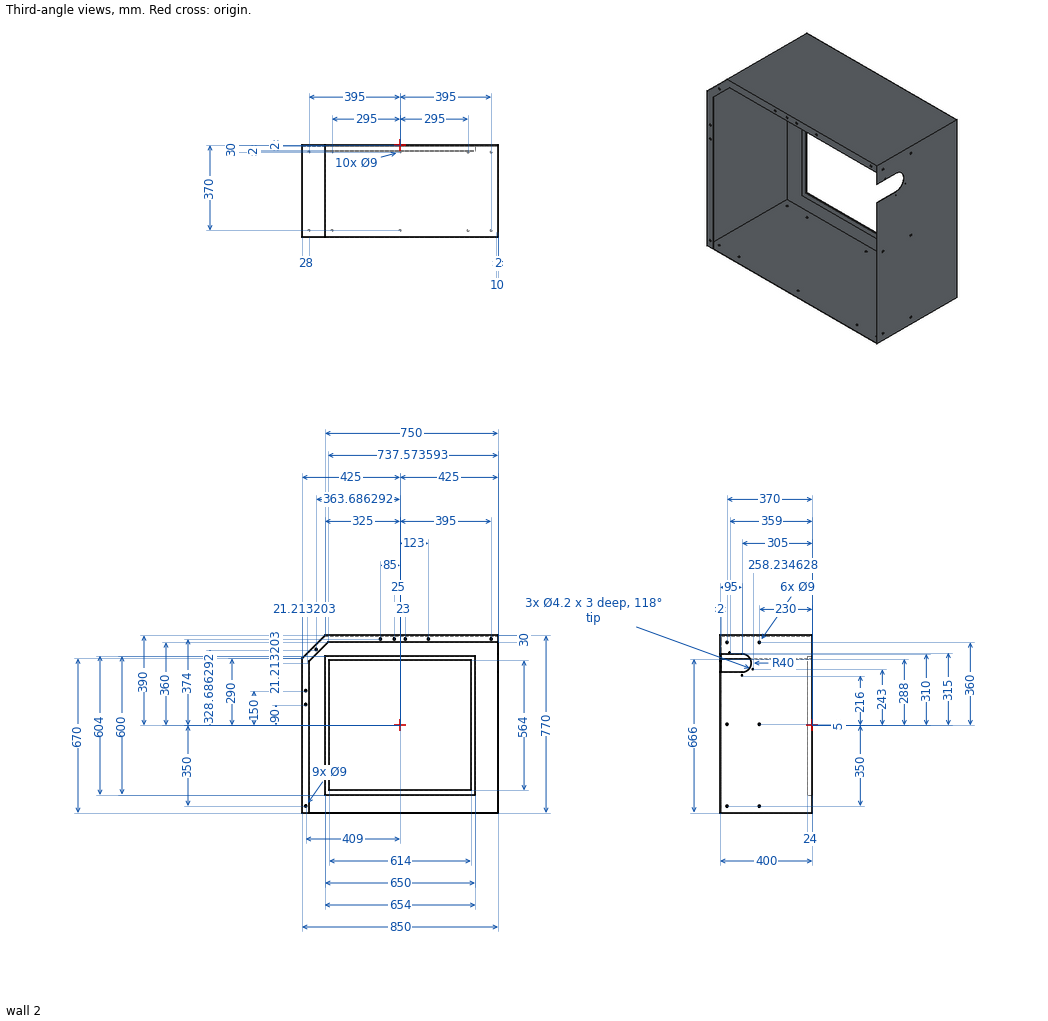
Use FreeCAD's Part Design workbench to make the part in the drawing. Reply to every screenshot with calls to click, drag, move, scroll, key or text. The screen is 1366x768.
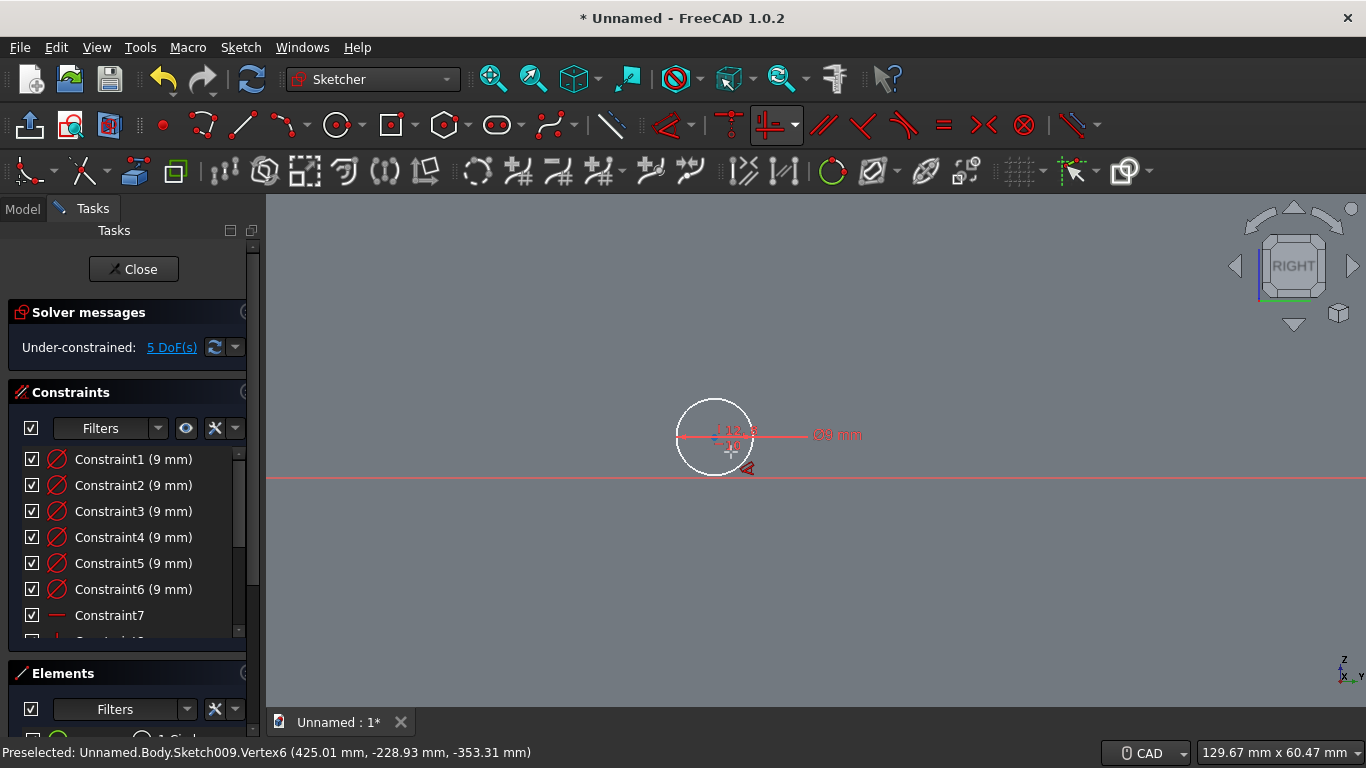
click(715, 437)
click(657, 458)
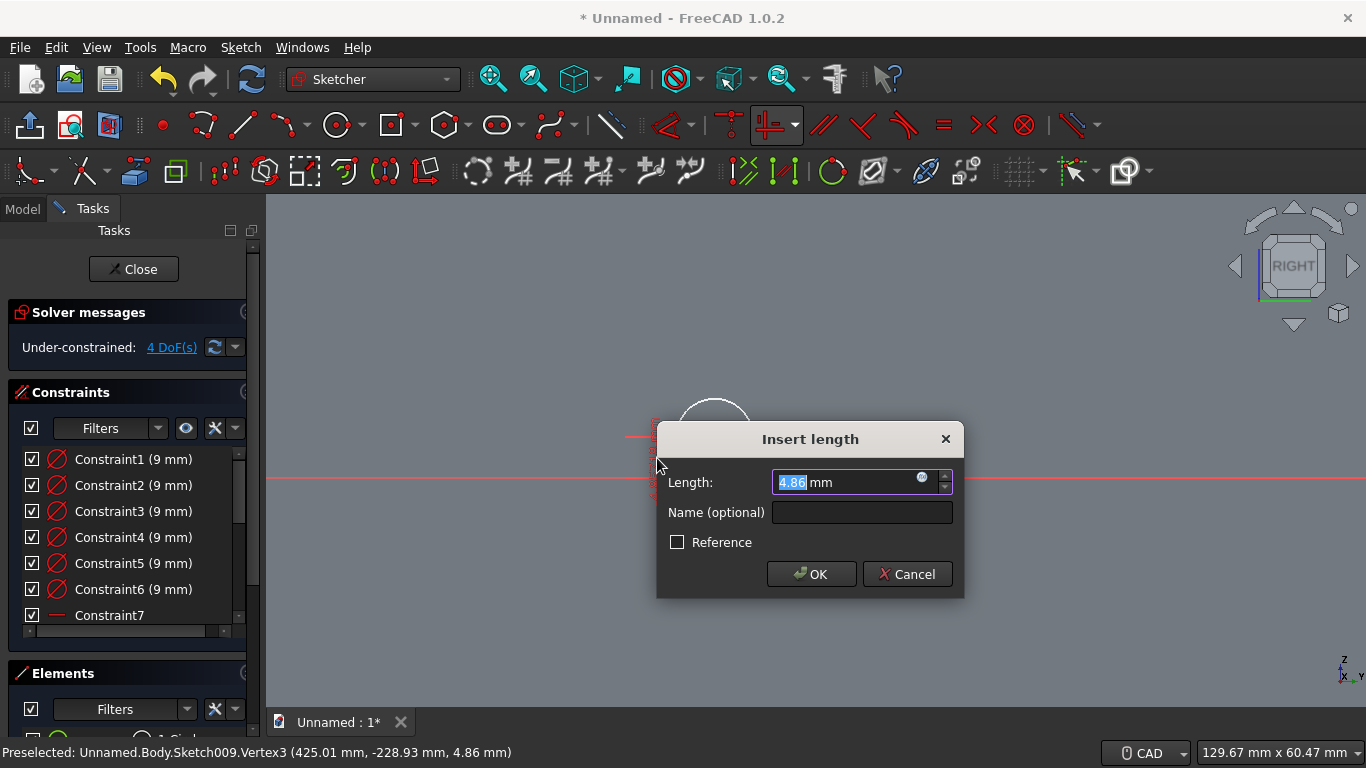
text(5)
key(Return)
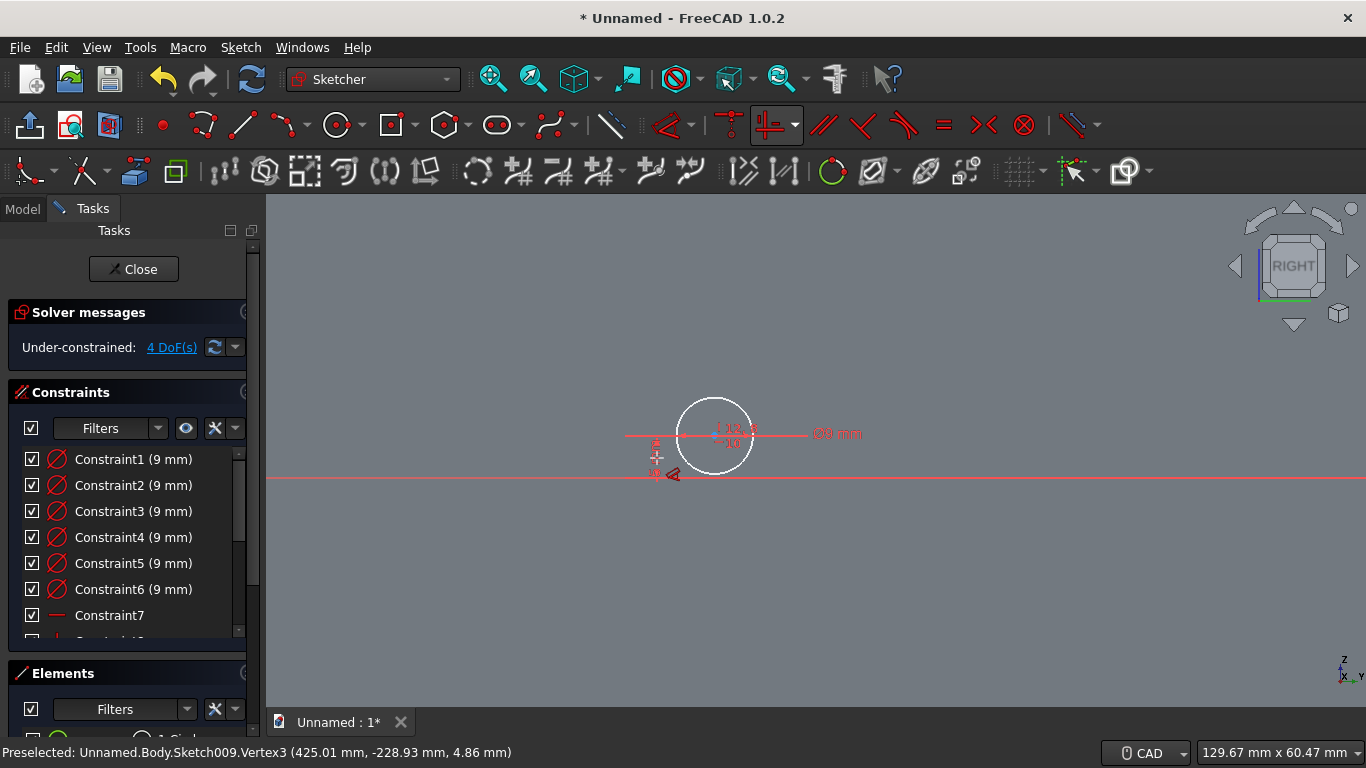
scroll(731, 451, down, 15)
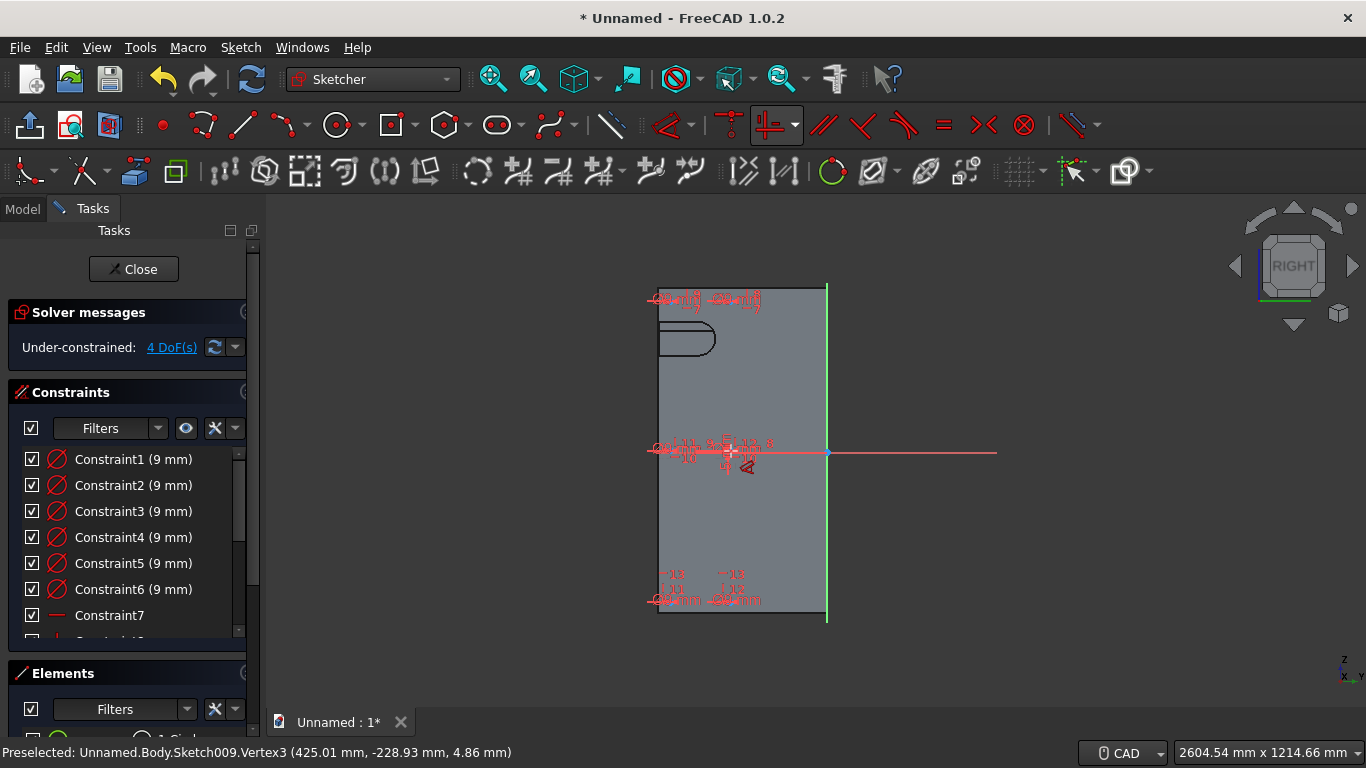
click(731, 301)
click(779, 267)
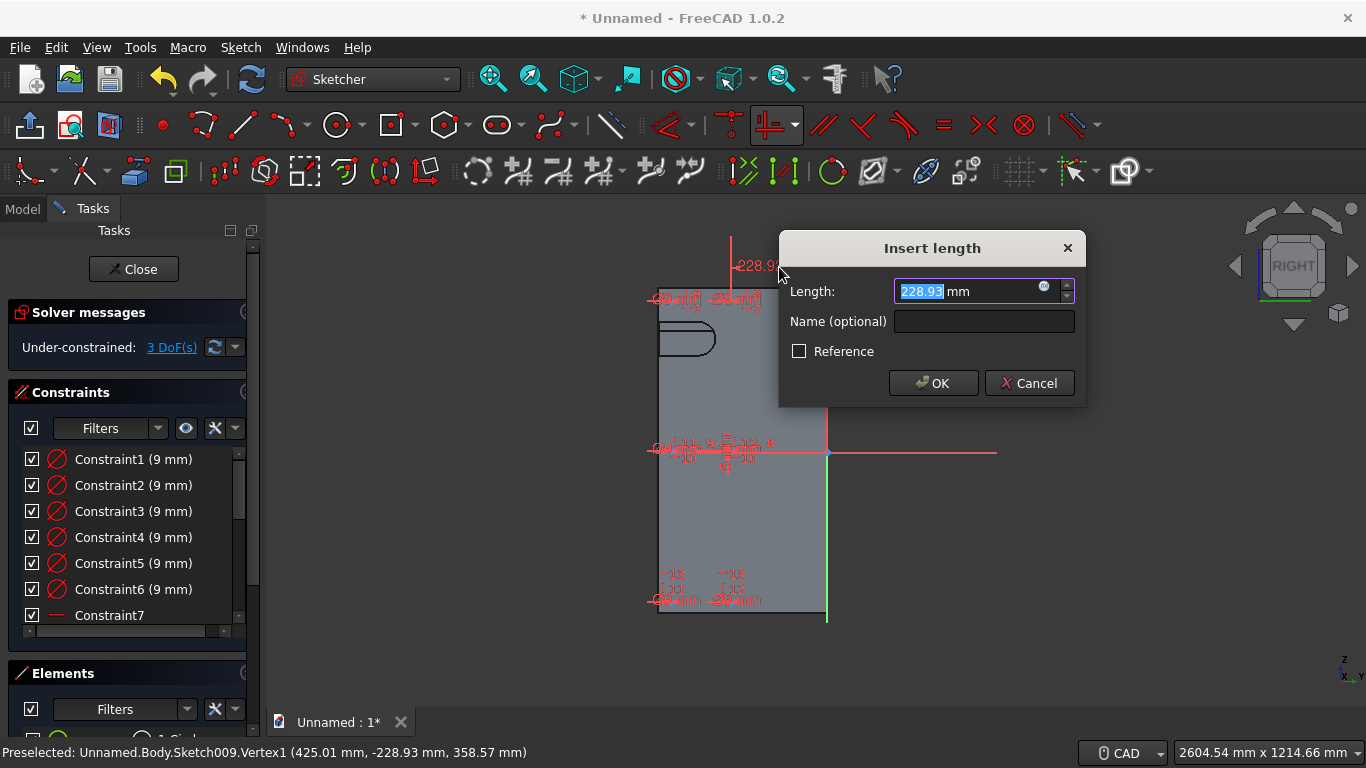
text(230)
key(Return)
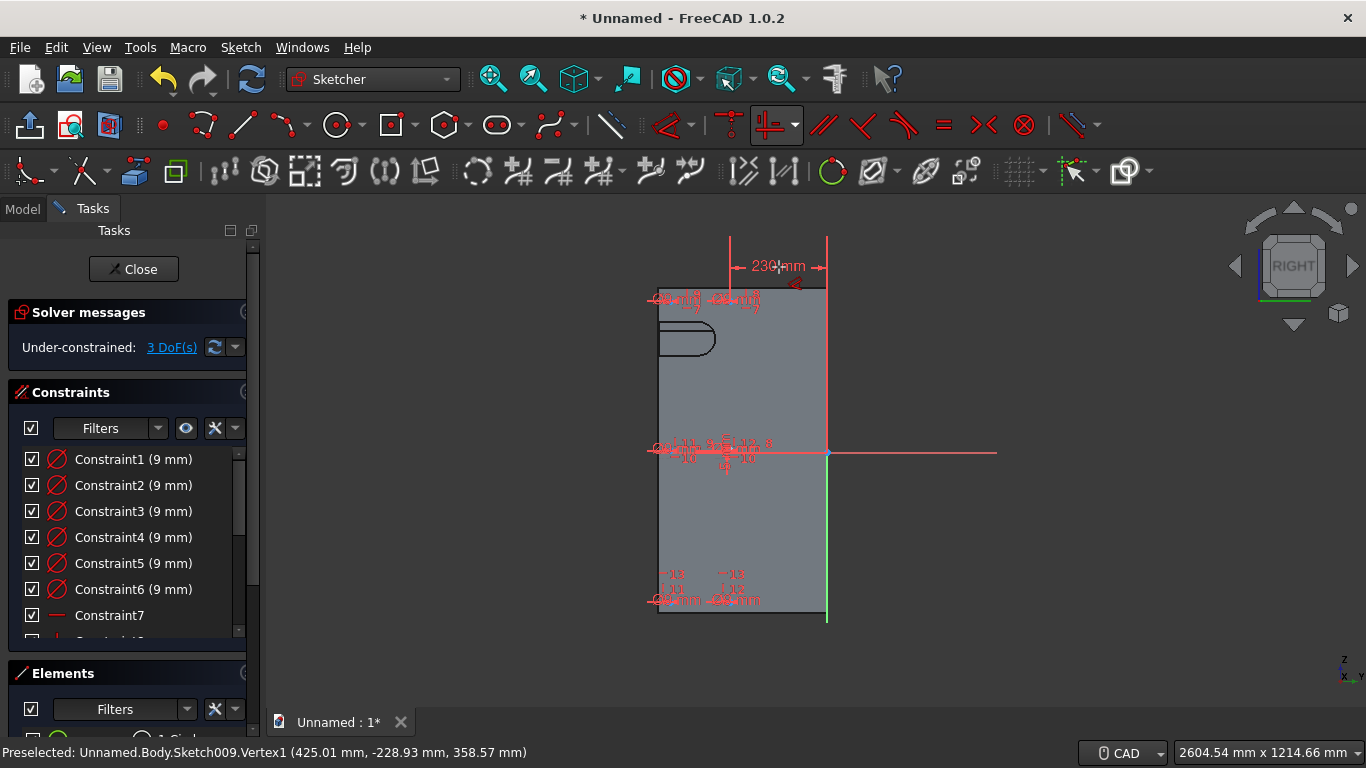
click(730, 301)
click(861, 377)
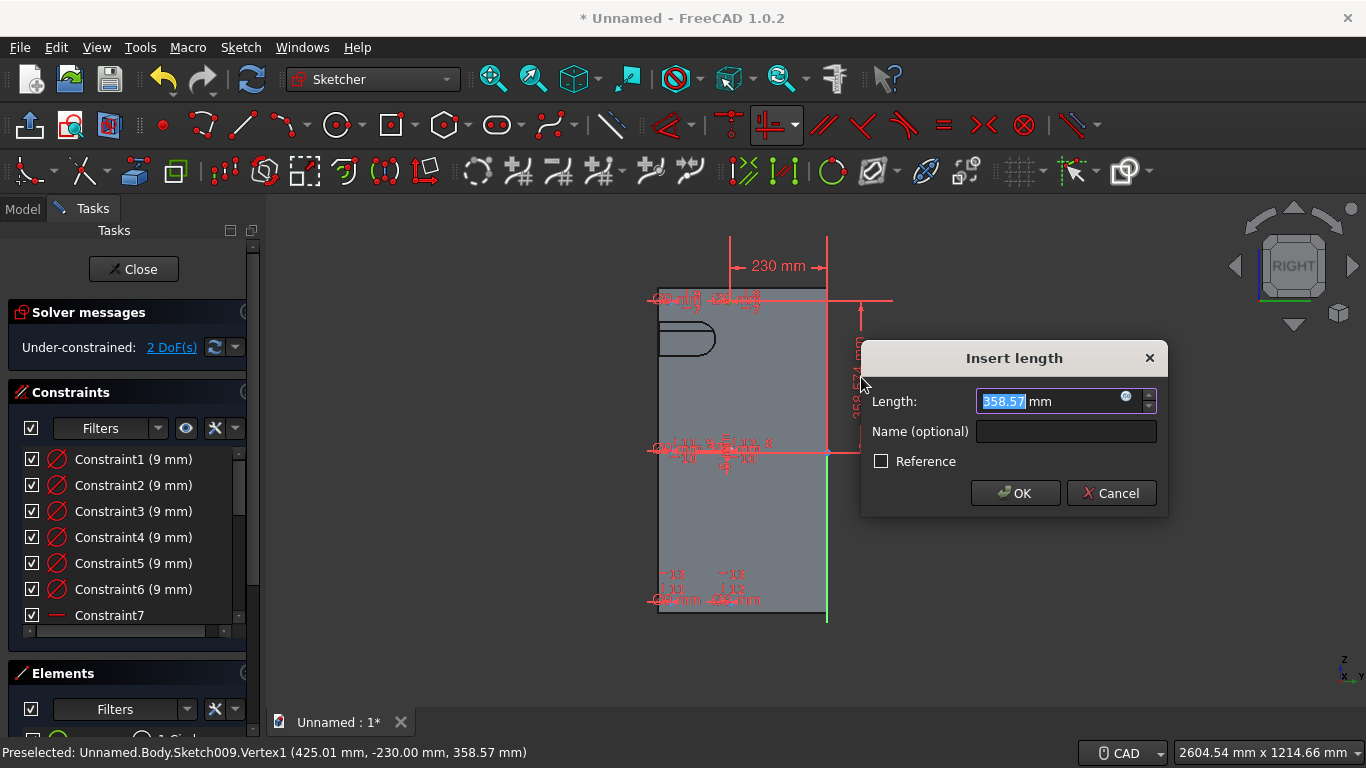
text(360)
key(Return)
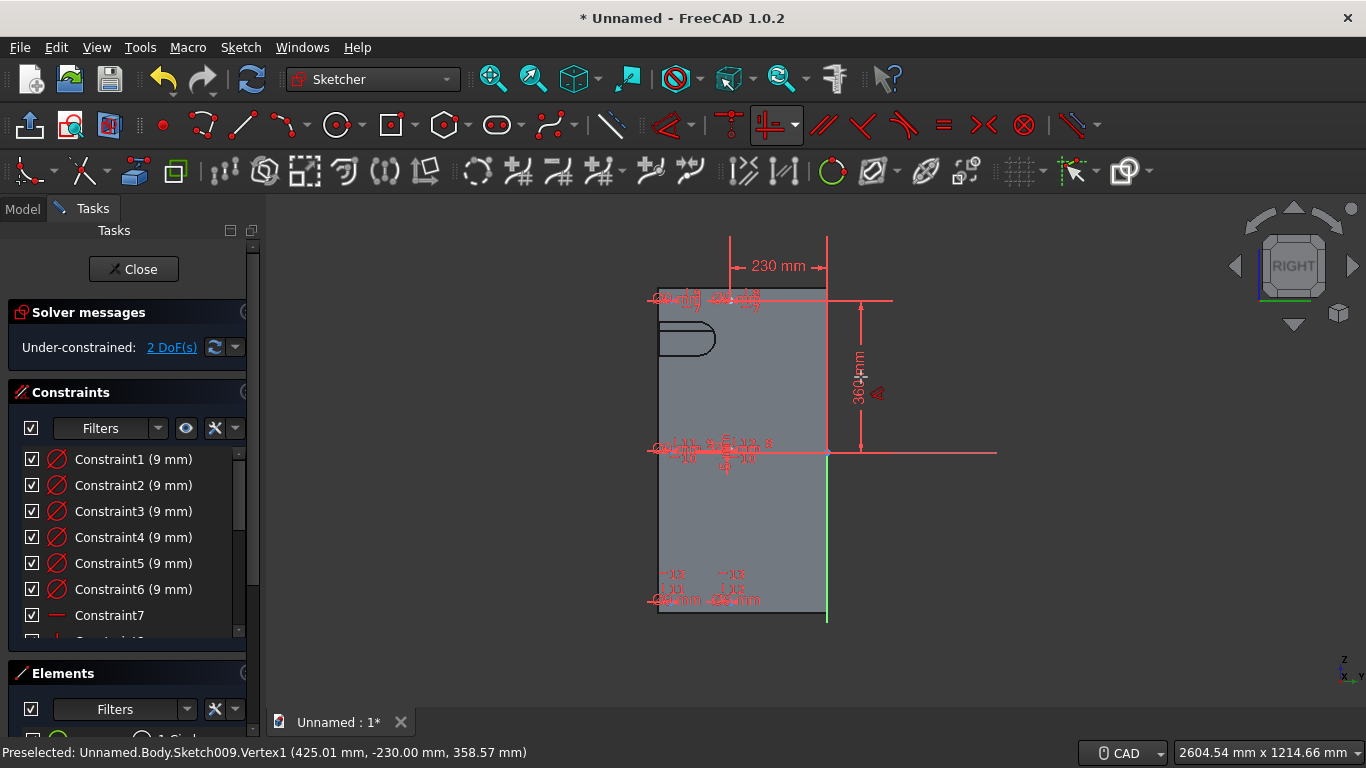
click(671, 301)
click(694, 267)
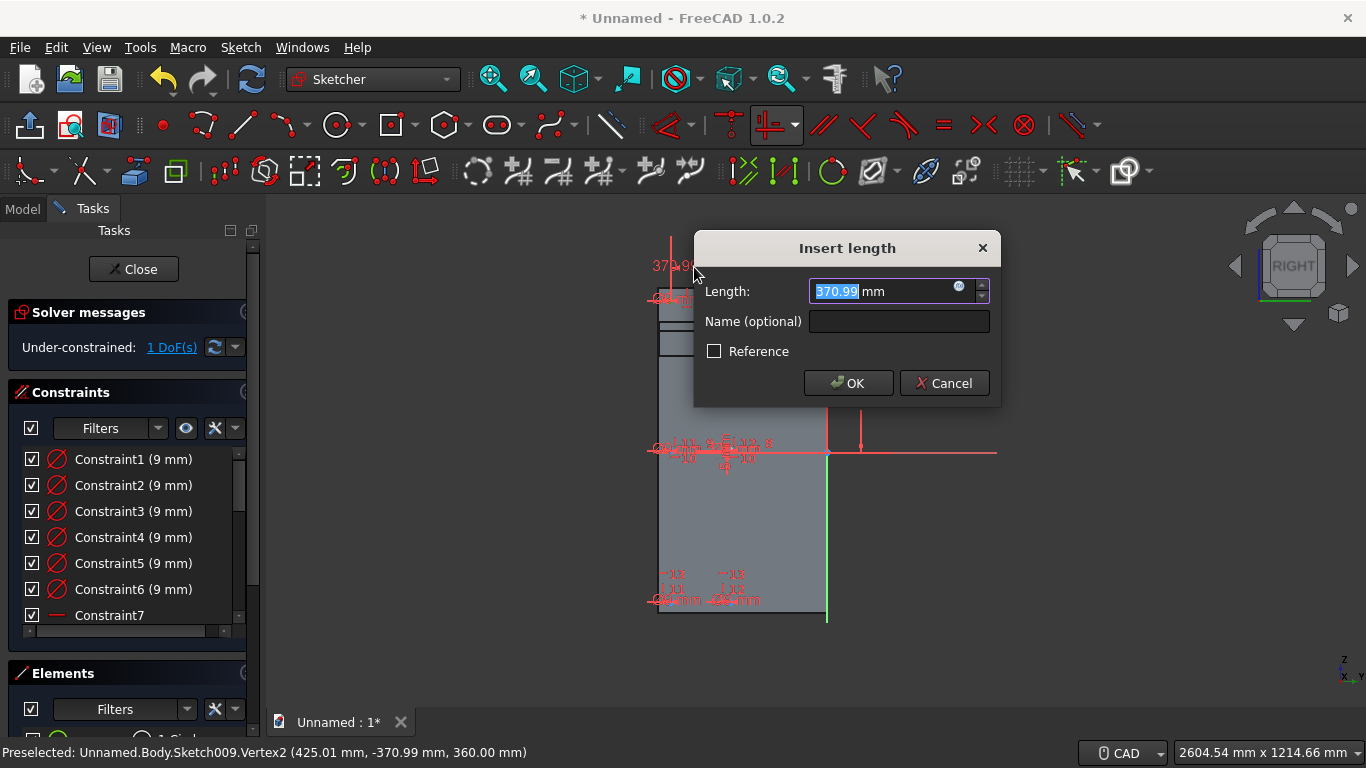
text(370)
key(Return)